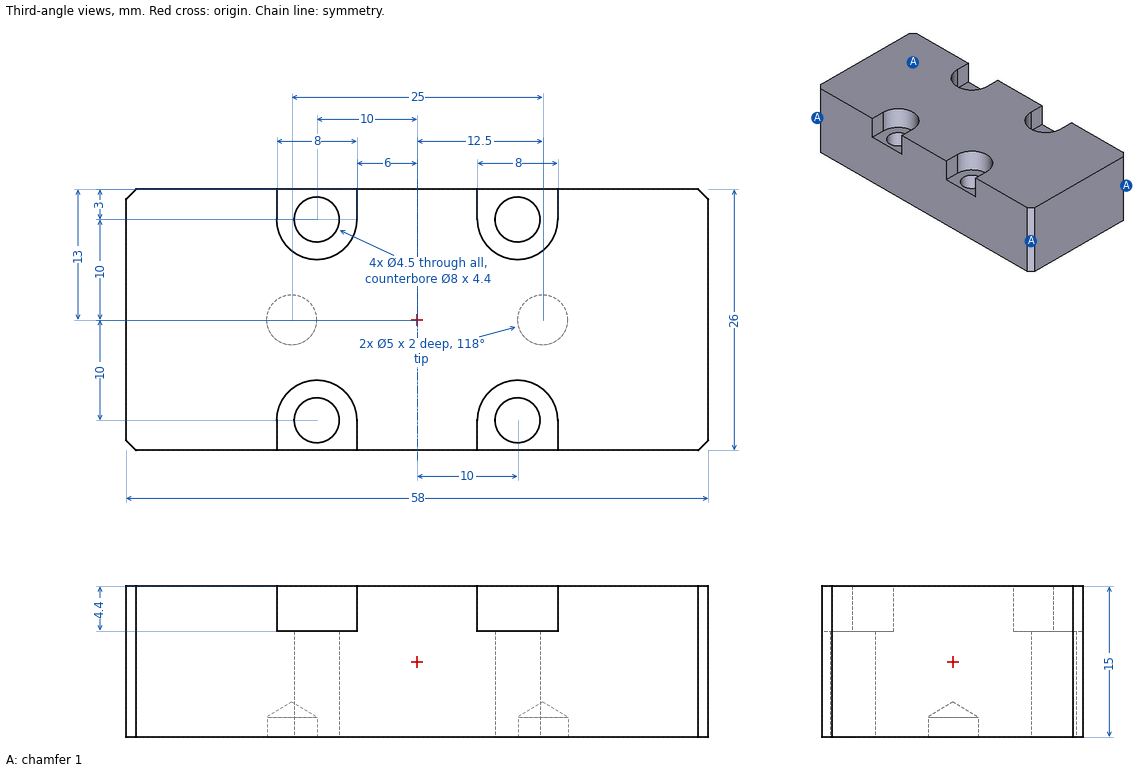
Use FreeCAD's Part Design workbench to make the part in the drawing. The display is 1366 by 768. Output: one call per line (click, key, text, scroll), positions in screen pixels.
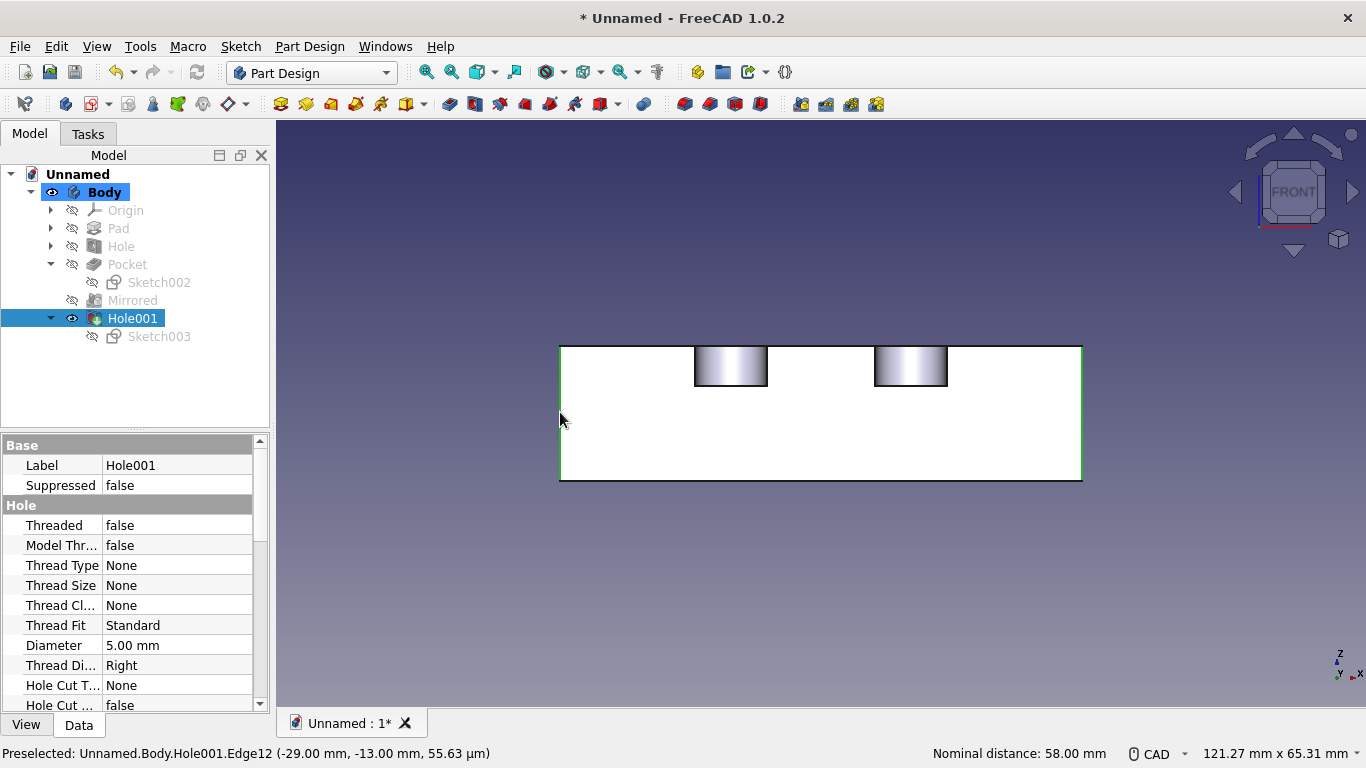
key(3)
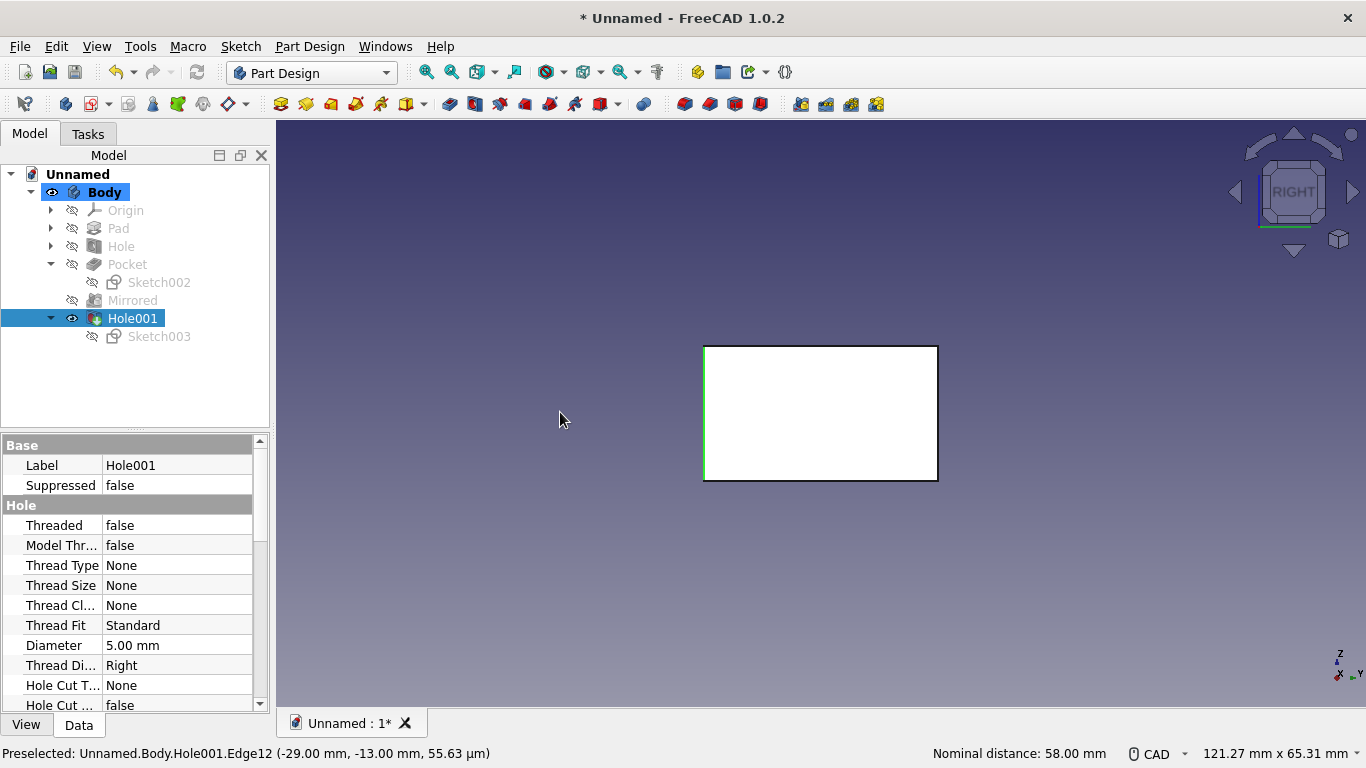
key(v)
key(f)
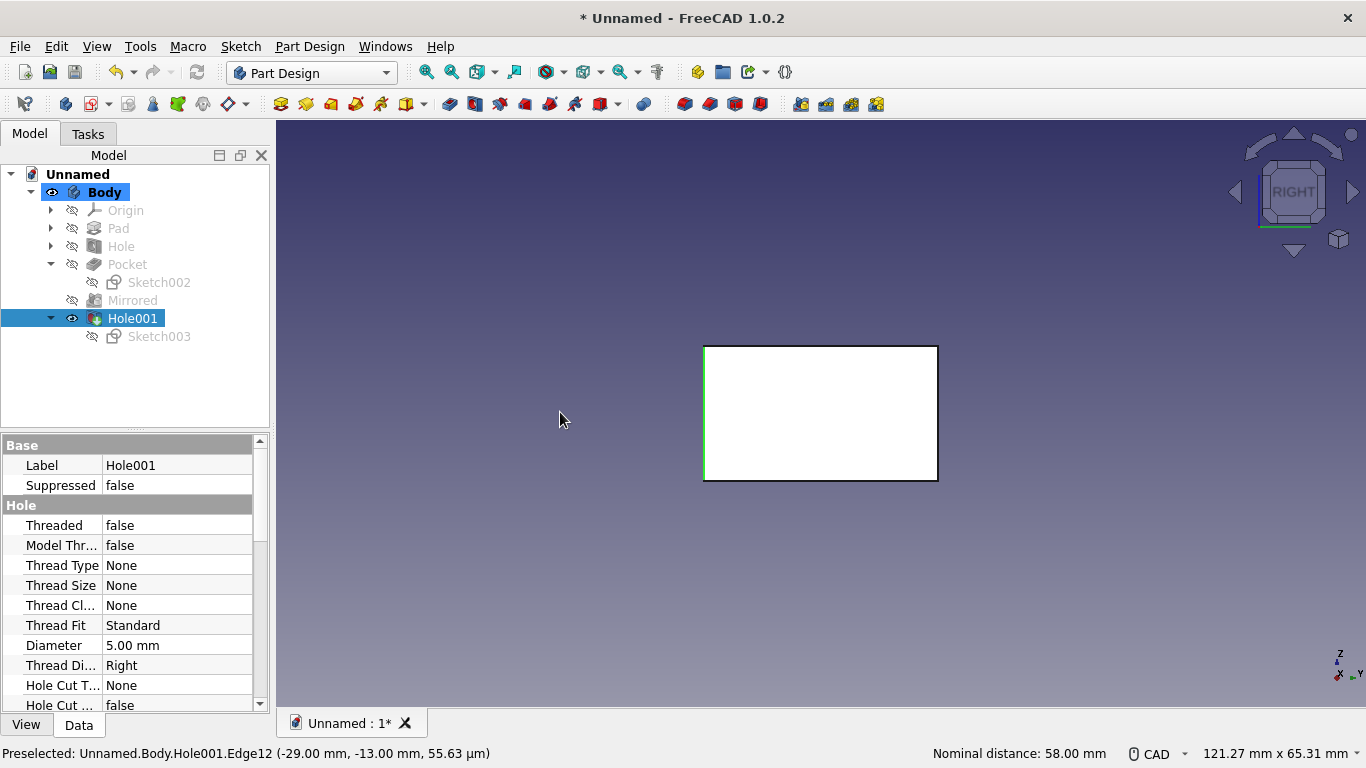
click(938, 412, ctrl)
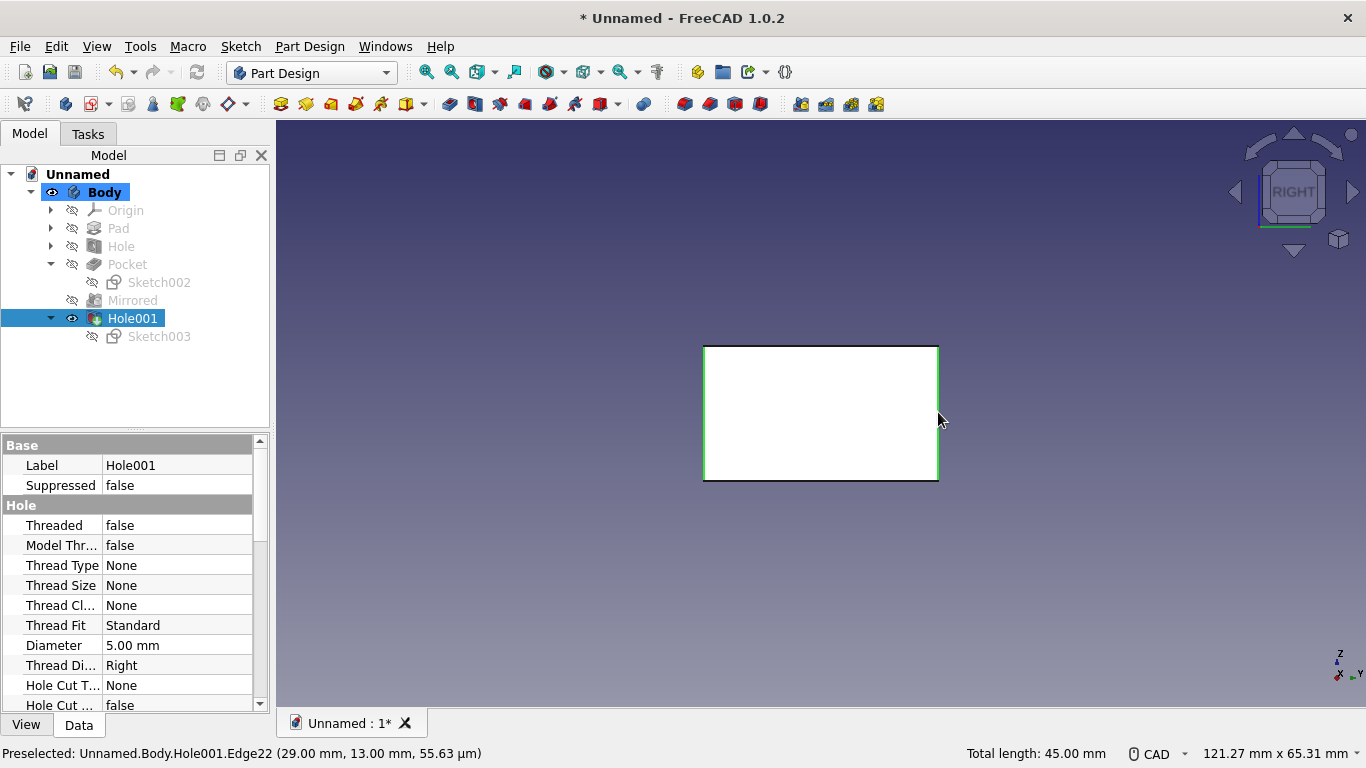
key(5)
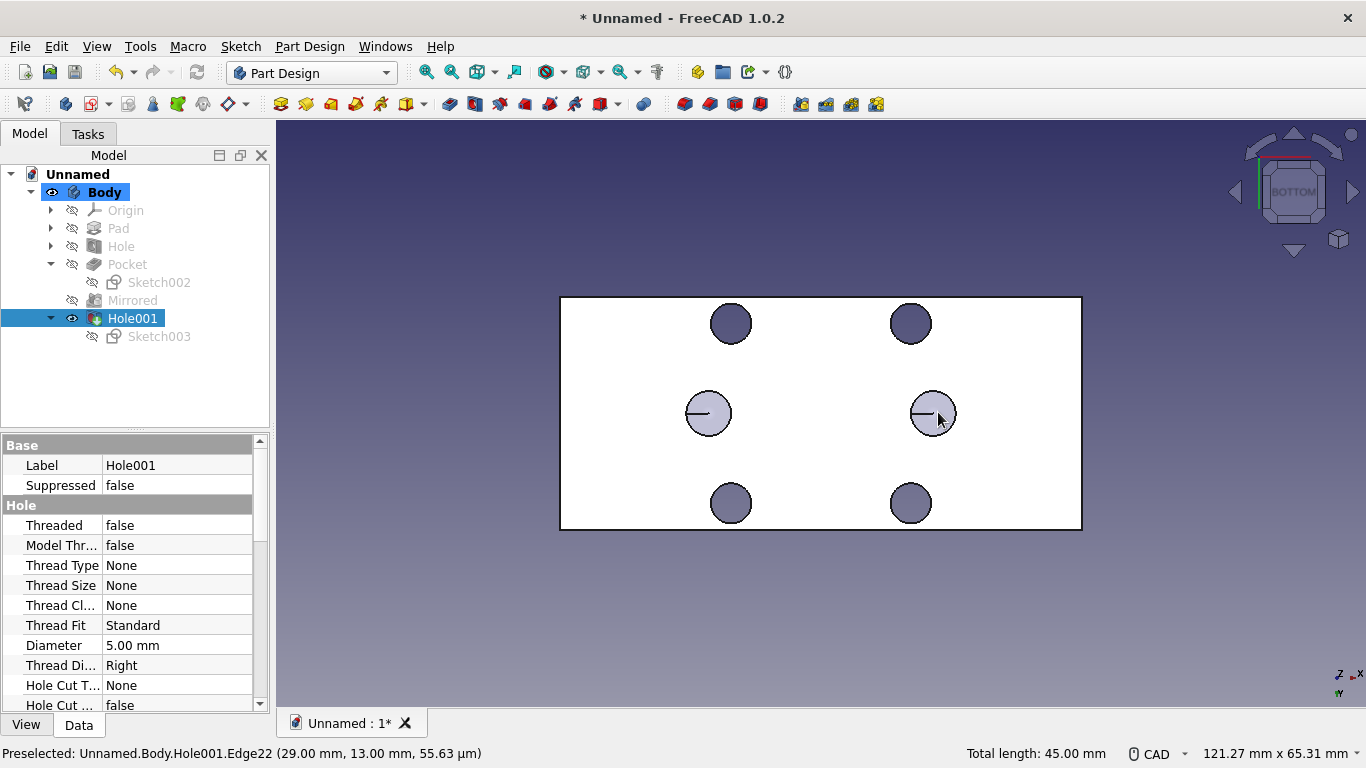
key(4)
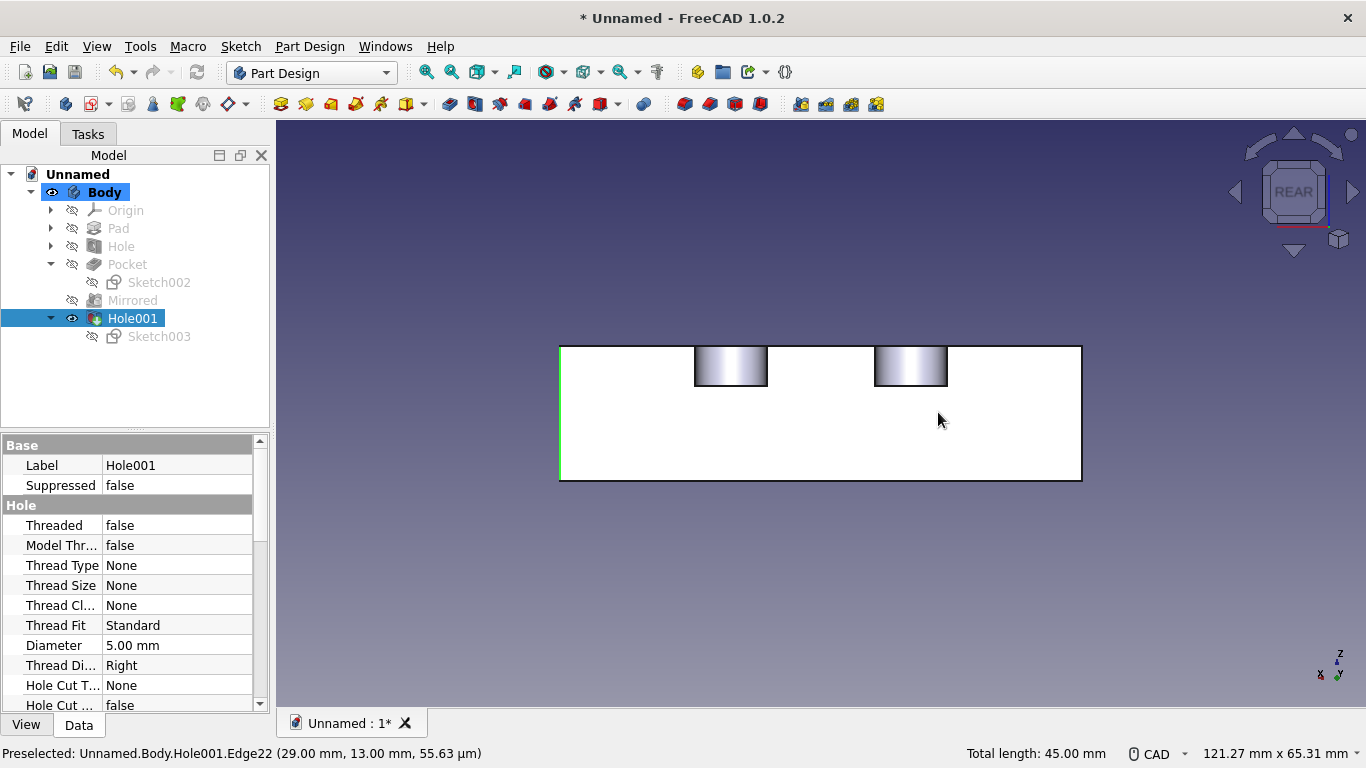
click(1082, 412, ctrl)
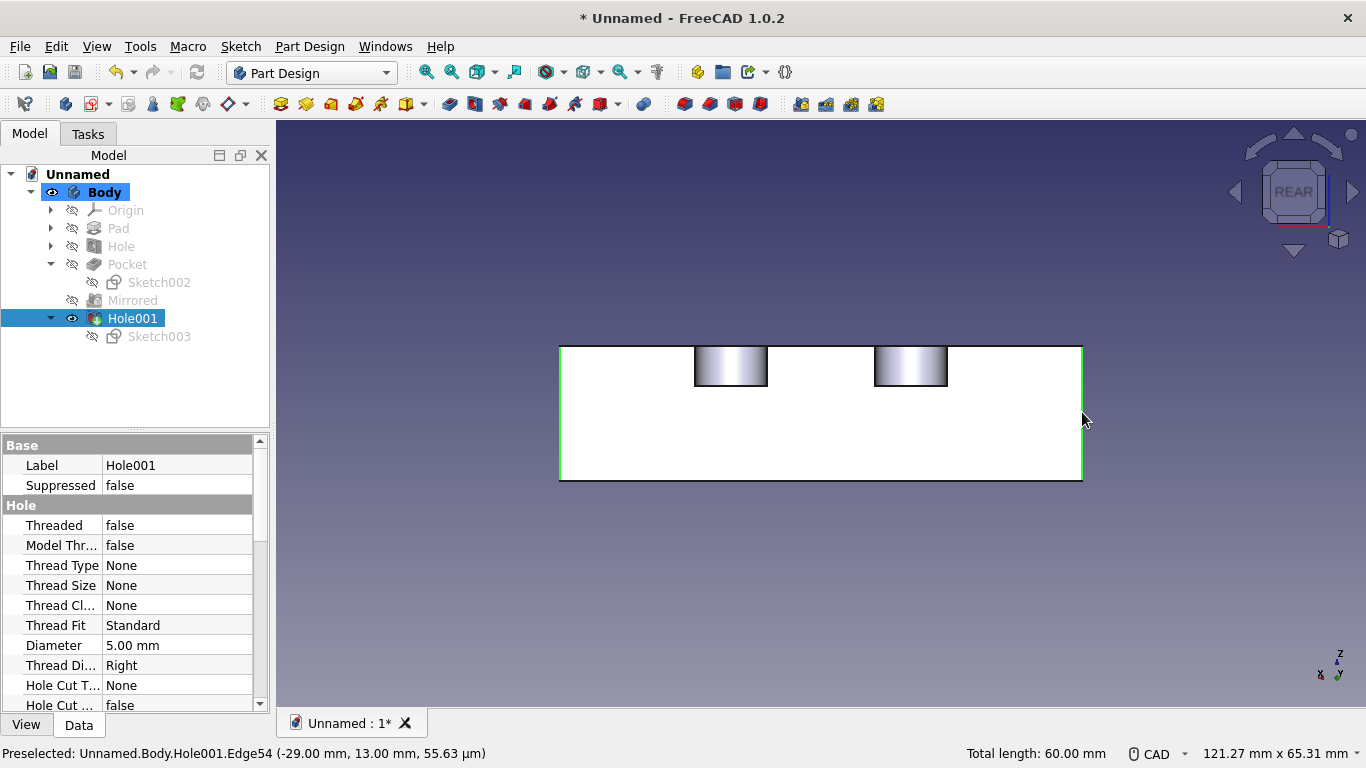
click(710, 104)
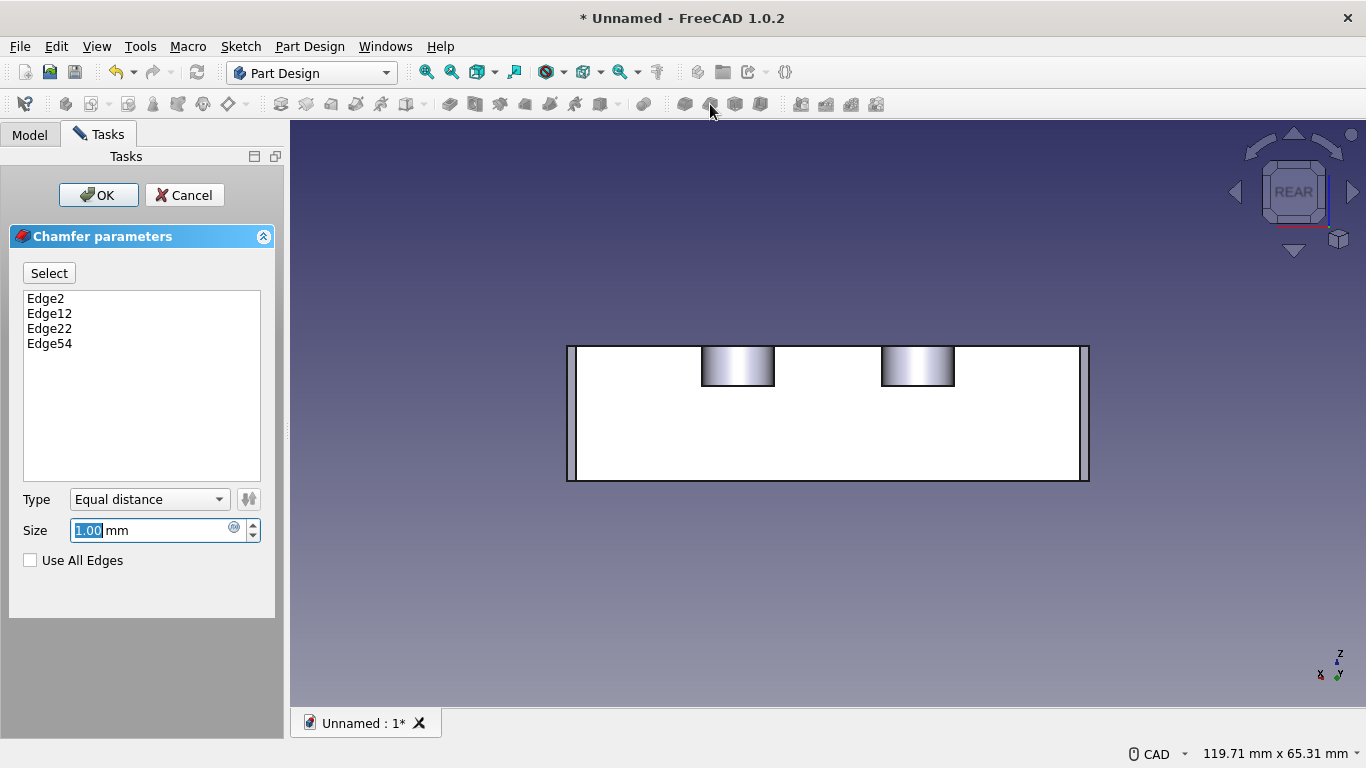
text(1)
key(Tab)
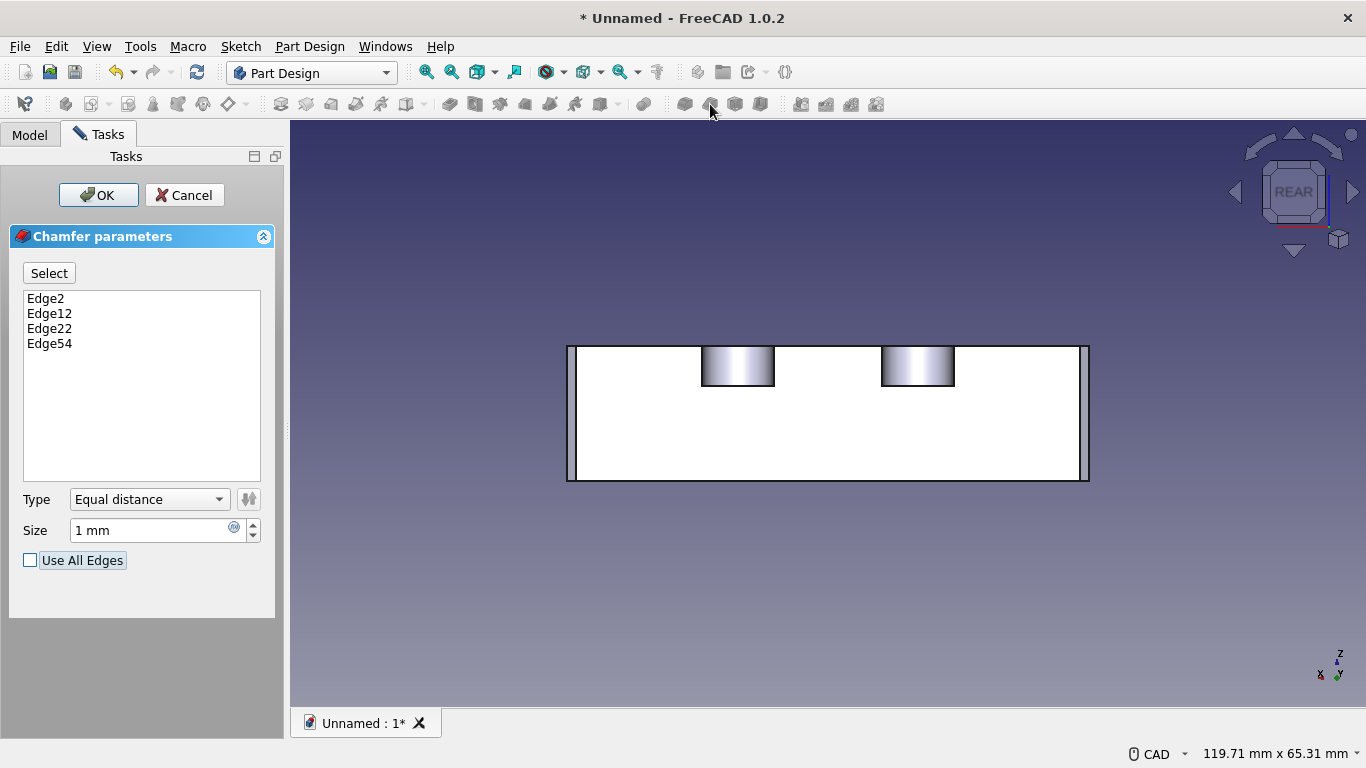
click(99, 195)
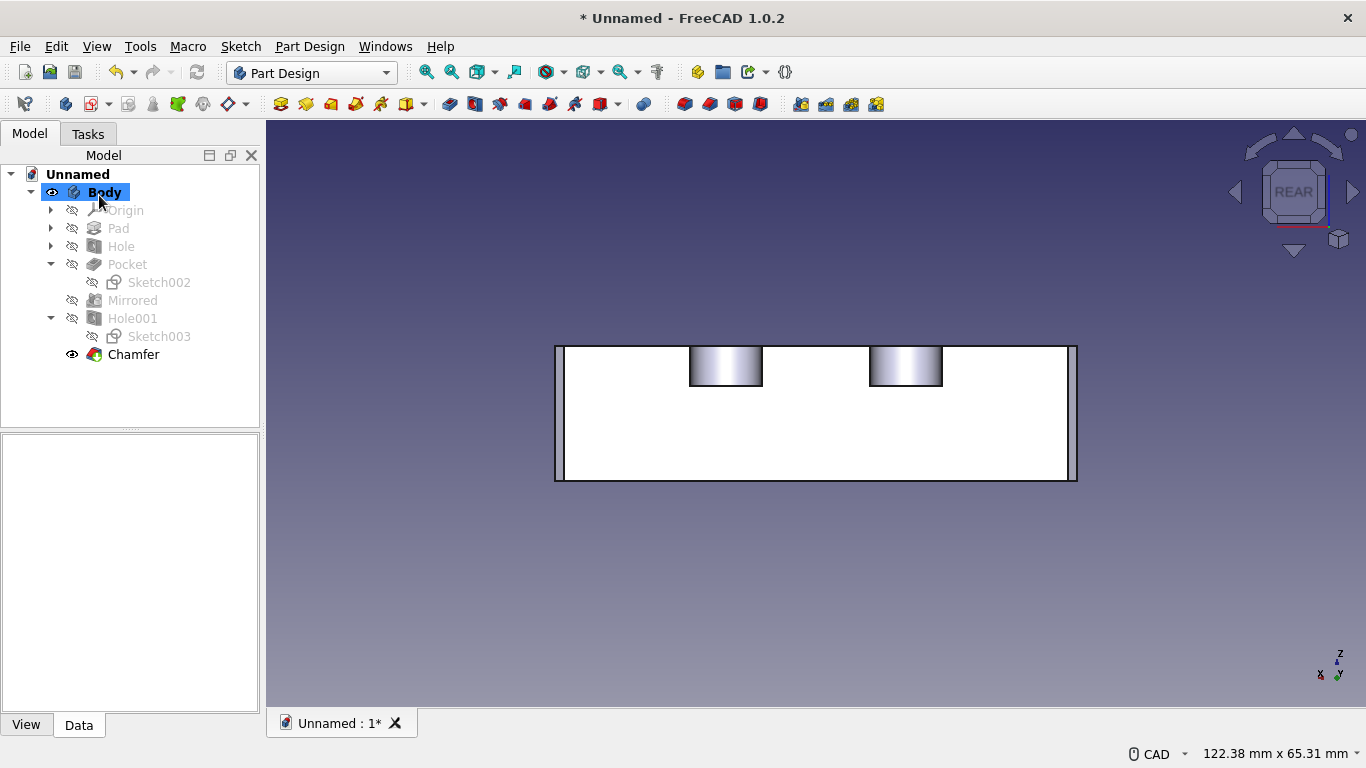
key(0)